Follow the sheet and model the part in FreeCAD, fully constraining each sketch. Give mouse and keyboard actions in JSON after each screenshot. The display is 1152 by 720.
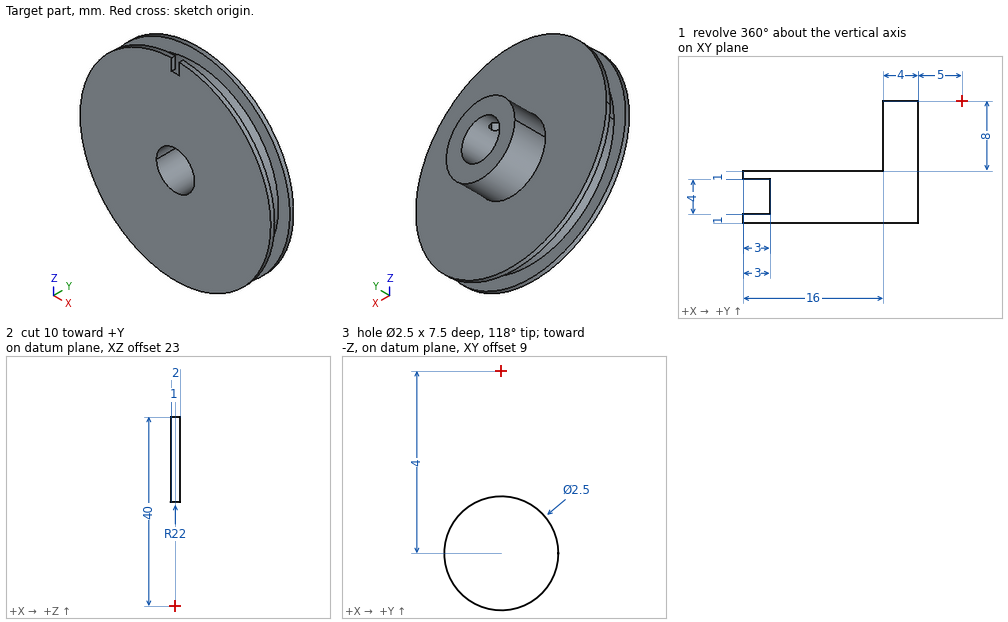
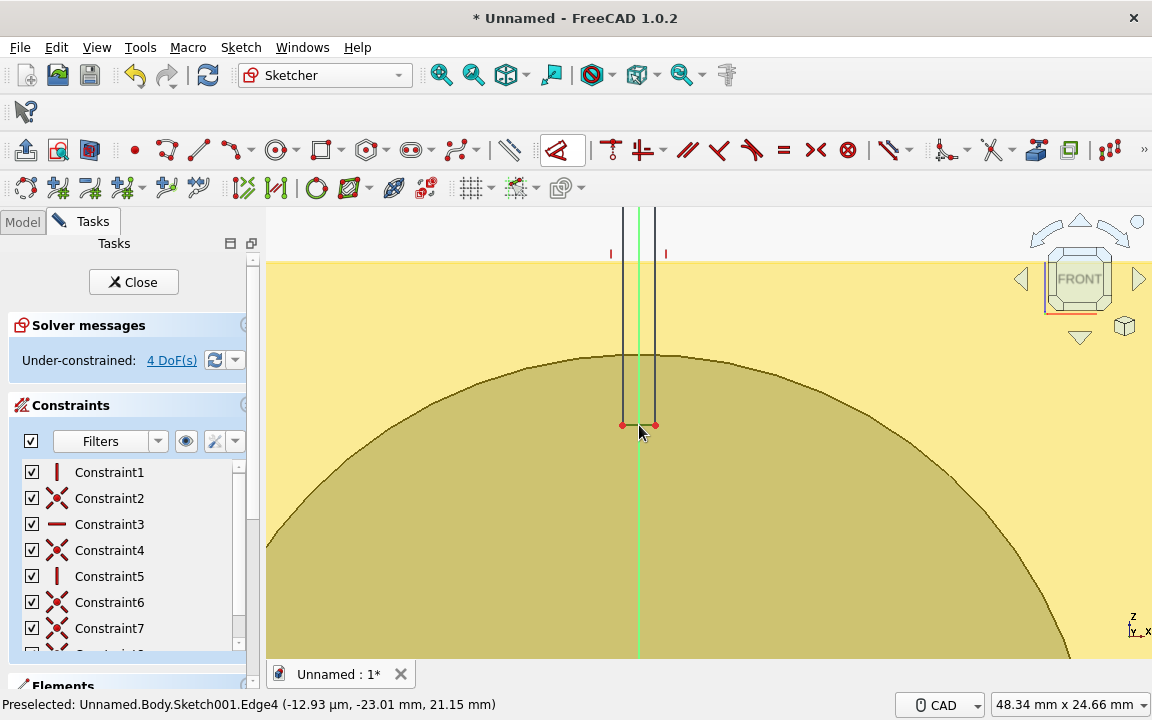
{"action": "key", "text": "k r"}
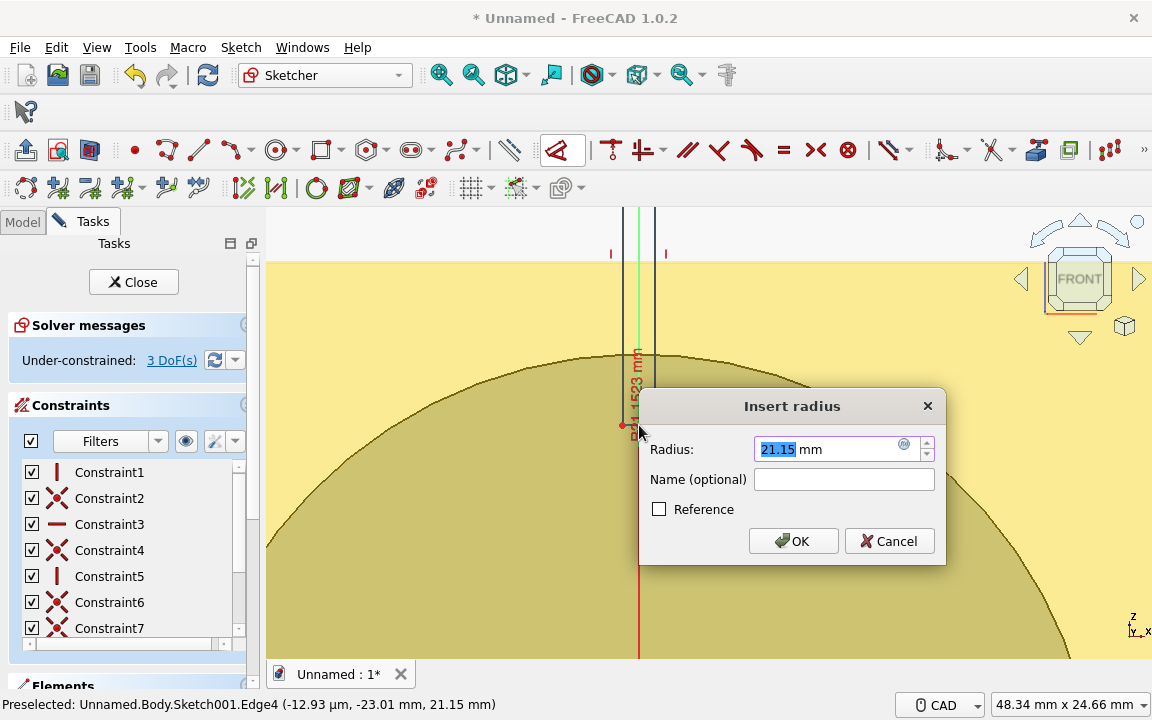
{"action": "type", "text": "22"}
{"action": "key", "text": "Return"}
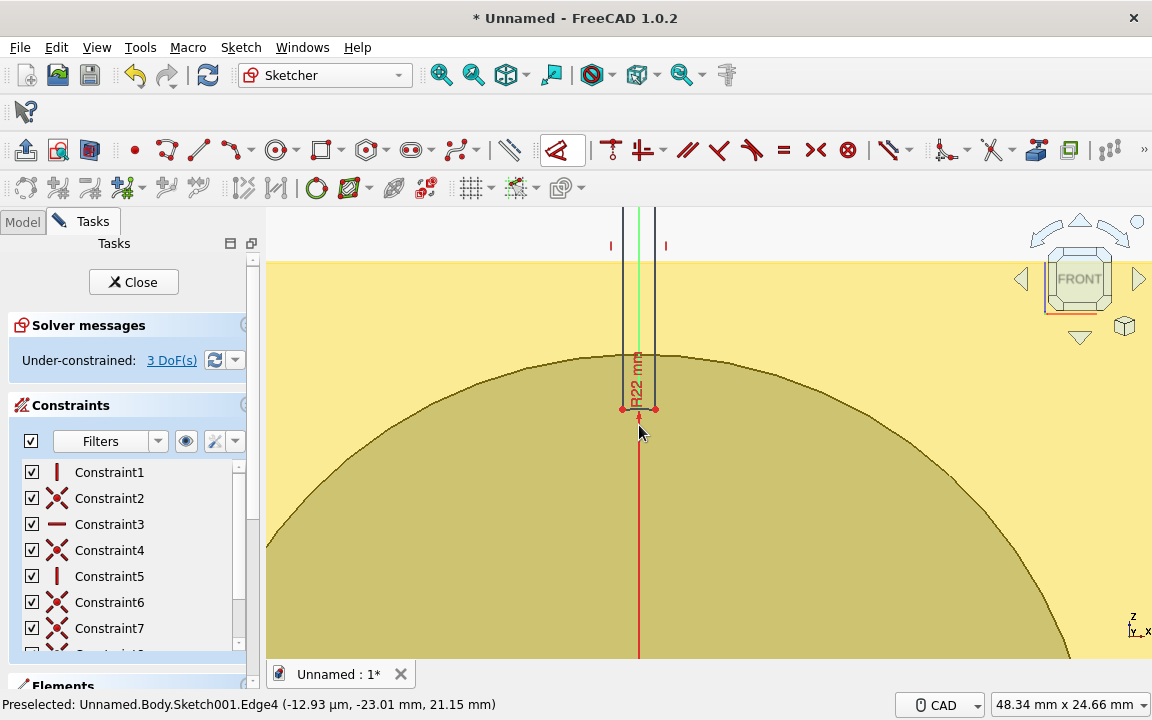
{"action": "scroll", "coordinate": [641, 425], "scroll_direction": "down", "scroll_amount": 5}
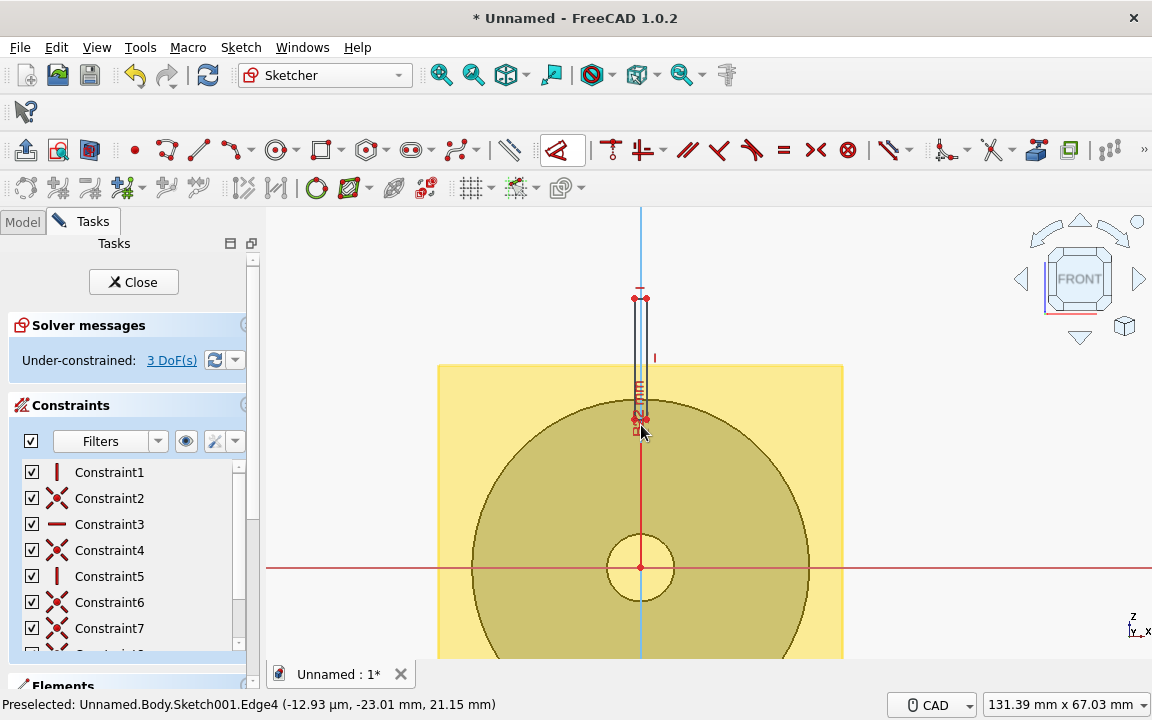
{"action": "scroll", "coordinate": [639, 299], "scroll_direction": "up", "scroll_amount": 6}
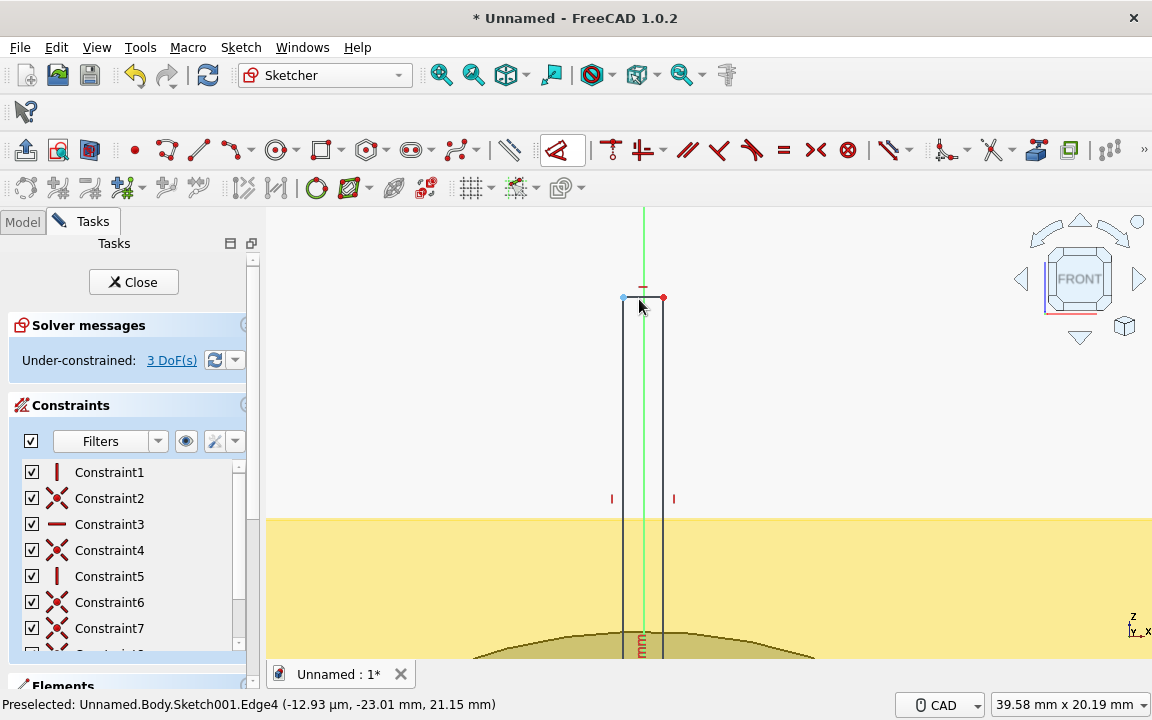
{"action": "left_click", "coordinate": [639, 297]}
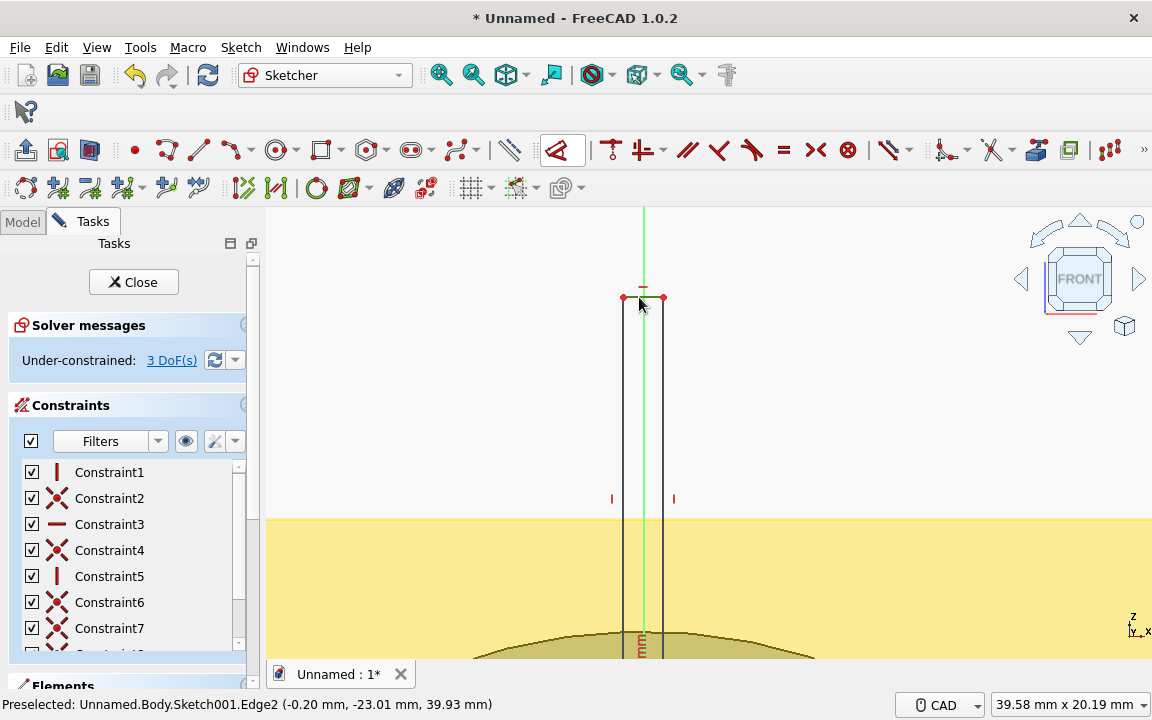
{"action": "left_click", "coordinate": [580, 150]}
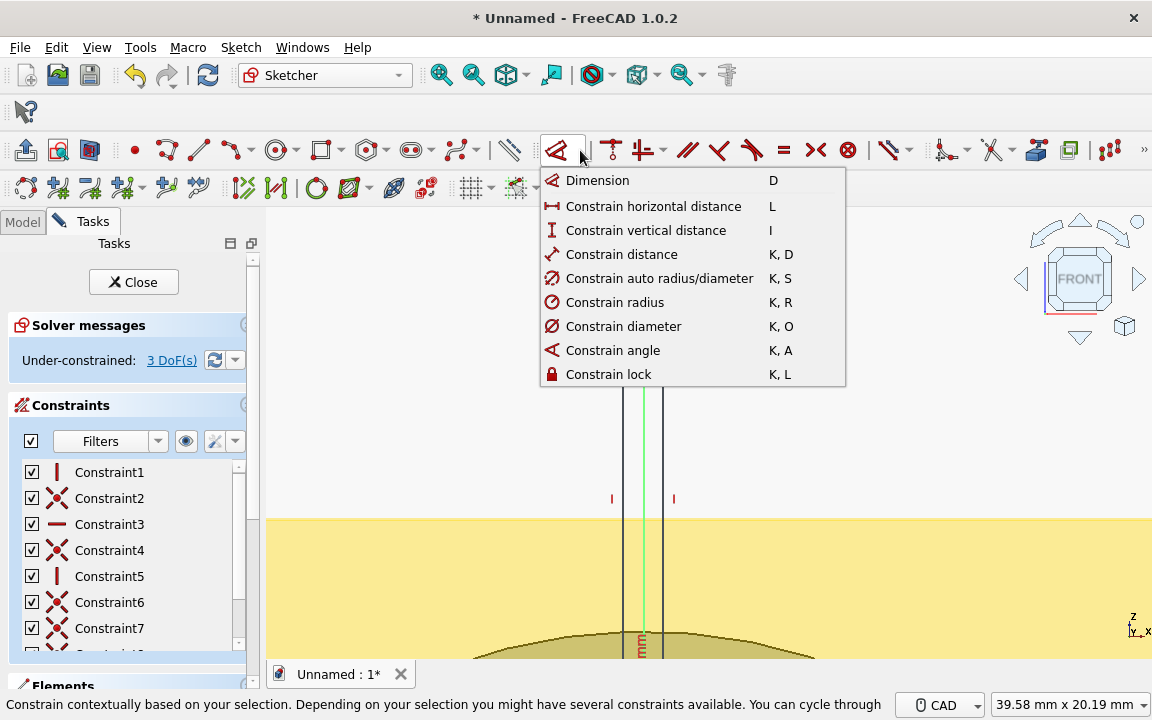
{"action": "left_click", "coordinate": [693, 206]}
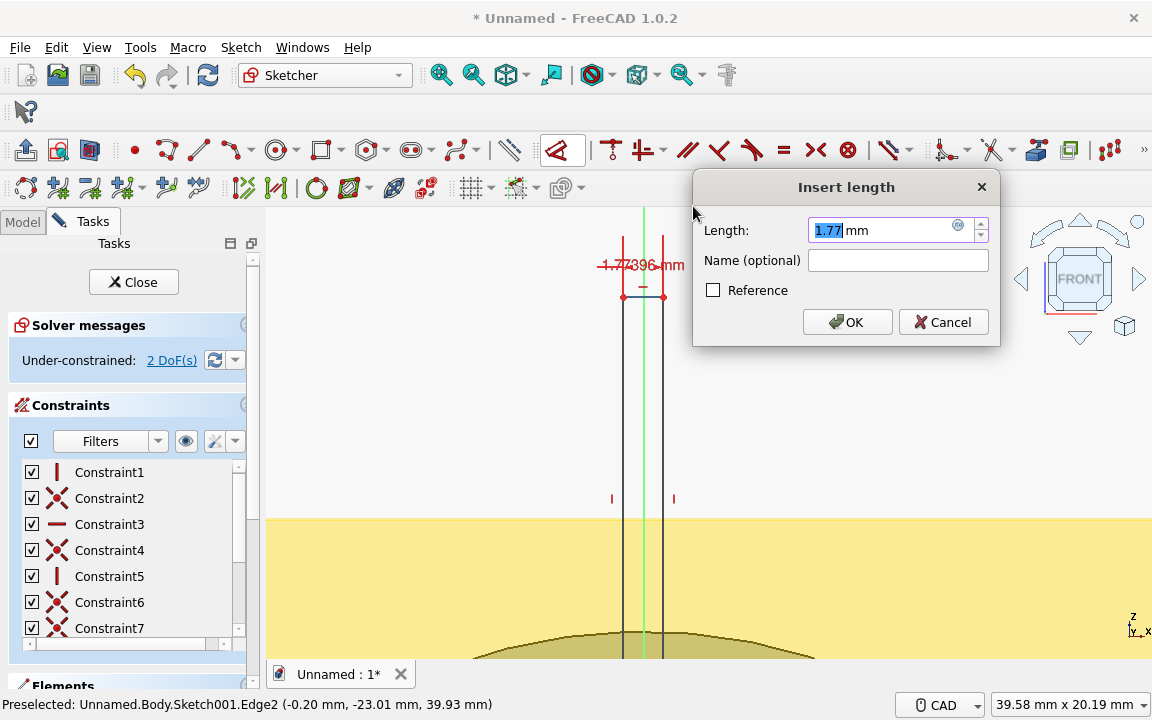
{"action": "type", "text": "2"}
{"action": "key", "text": "Return"}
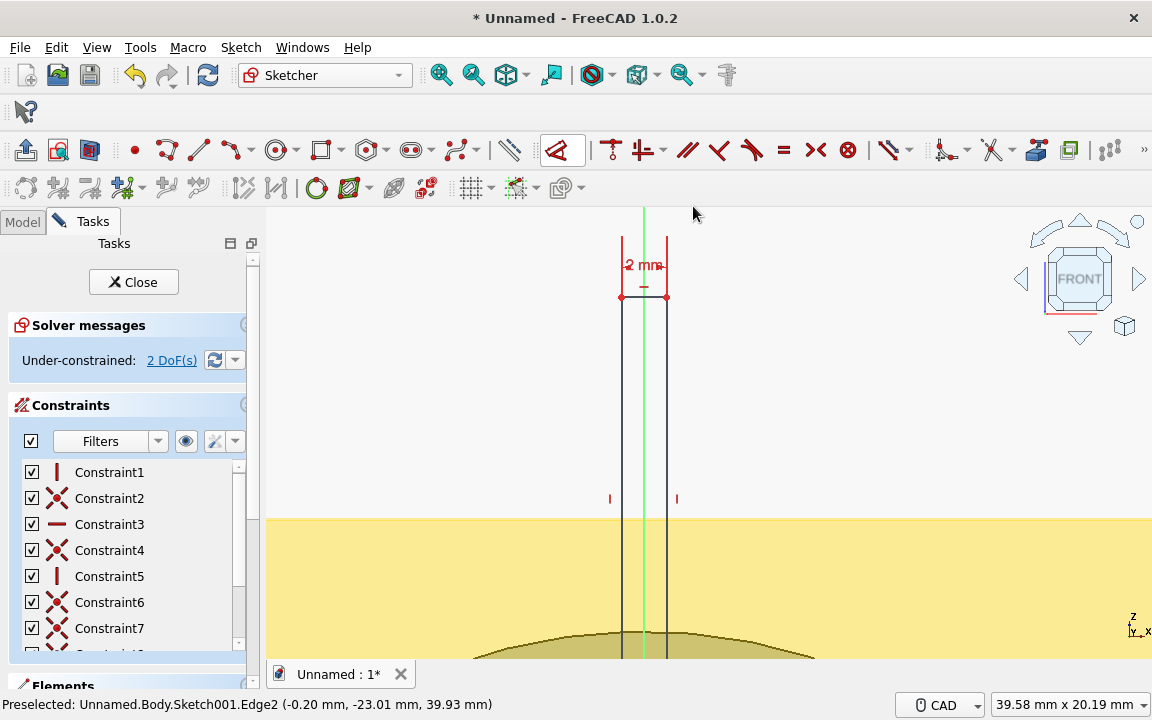
{"action": "scroll", "coordinate": [639, 299], "scroll_direction": "down", "scroll_amount": 6}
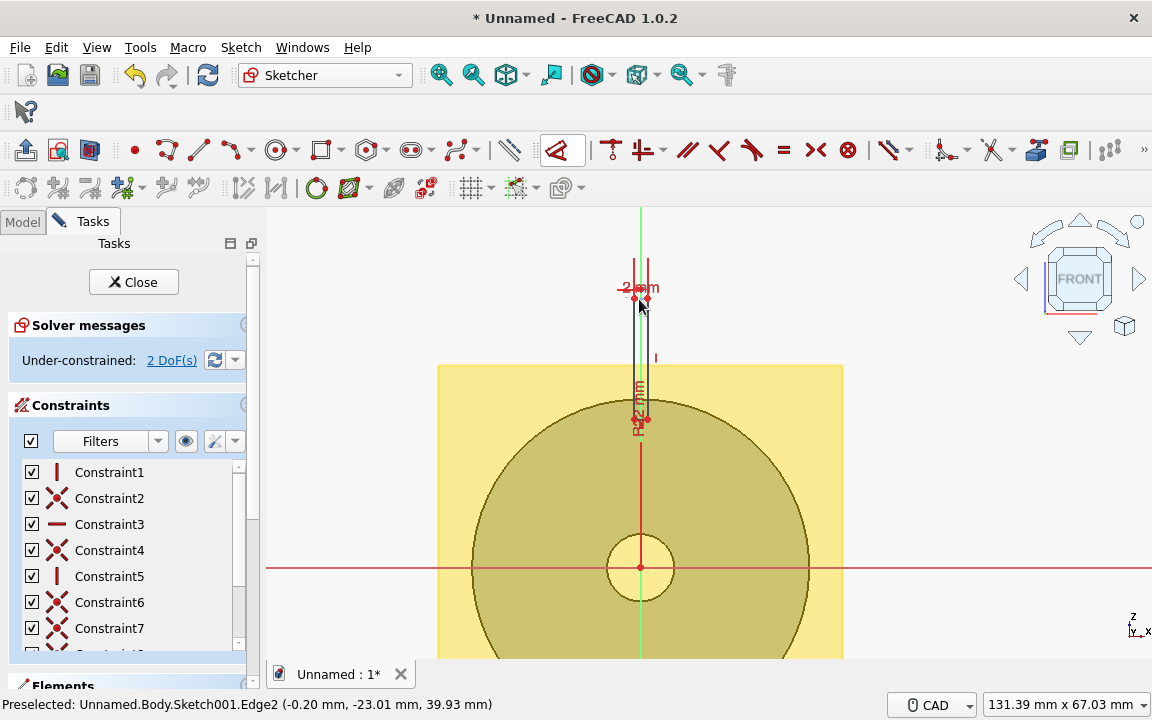
{"action": "scroll", "coordinate": [634, 420], "scroll_direction": "up", "scroll_amount": 9}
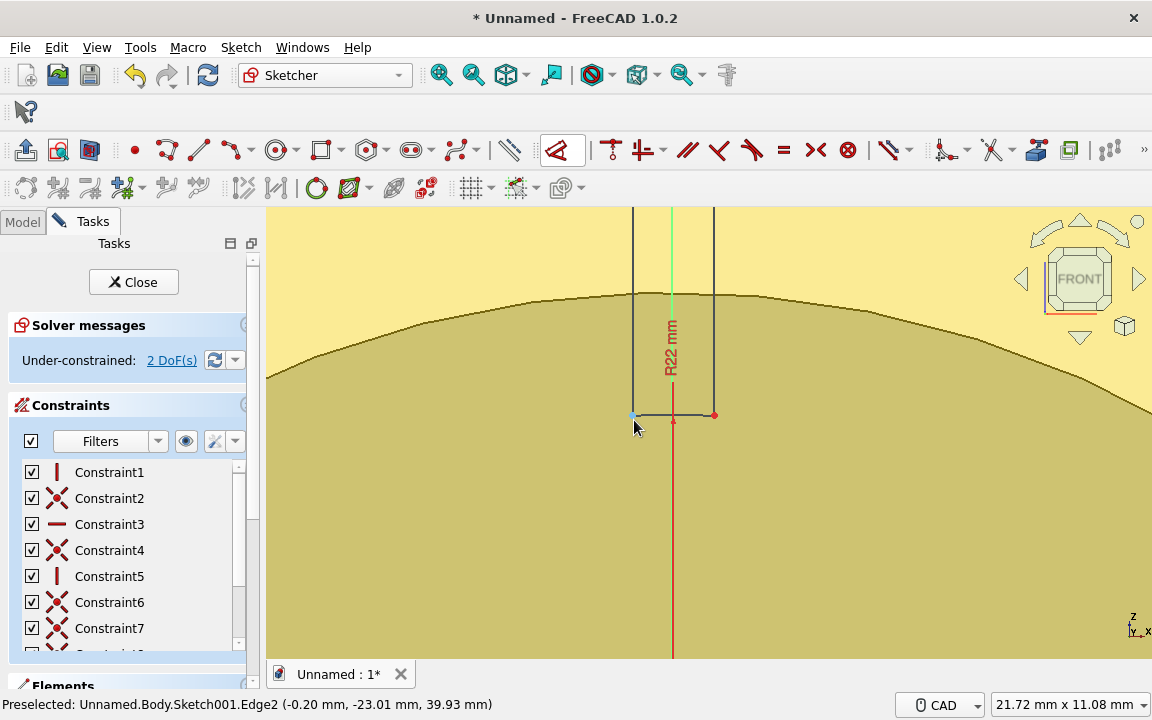
{"action": "left_click", "coordinate": [633, 416]}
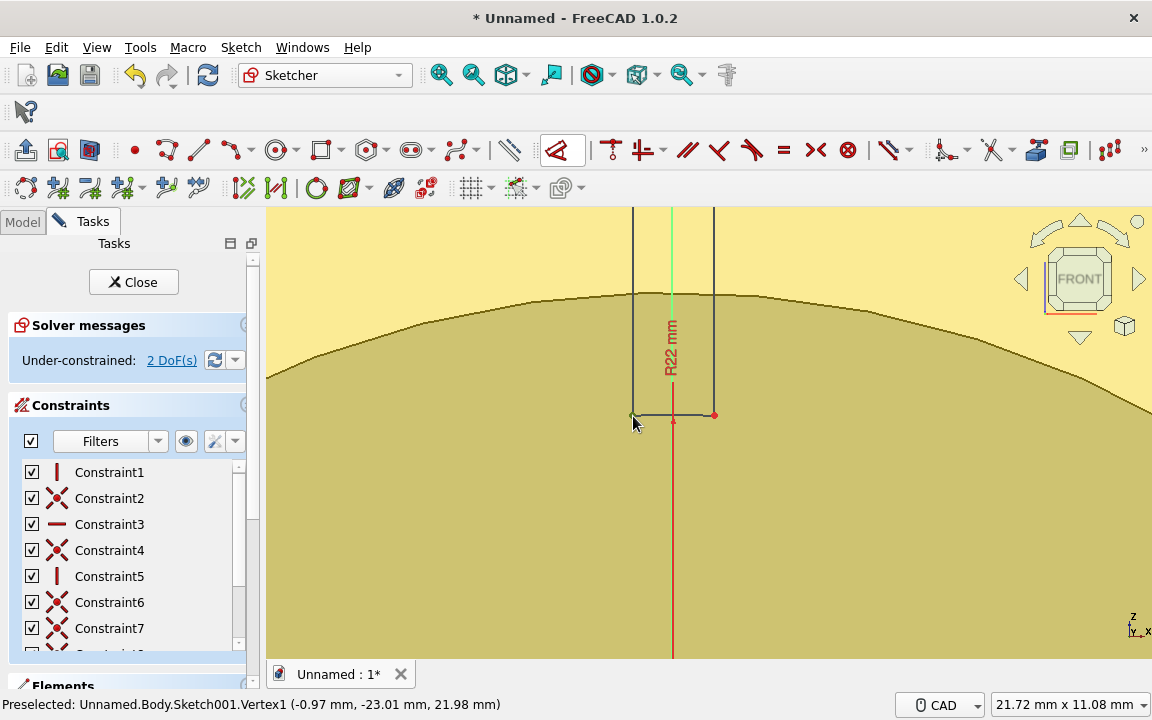
{"action": "key", "text": "l"}